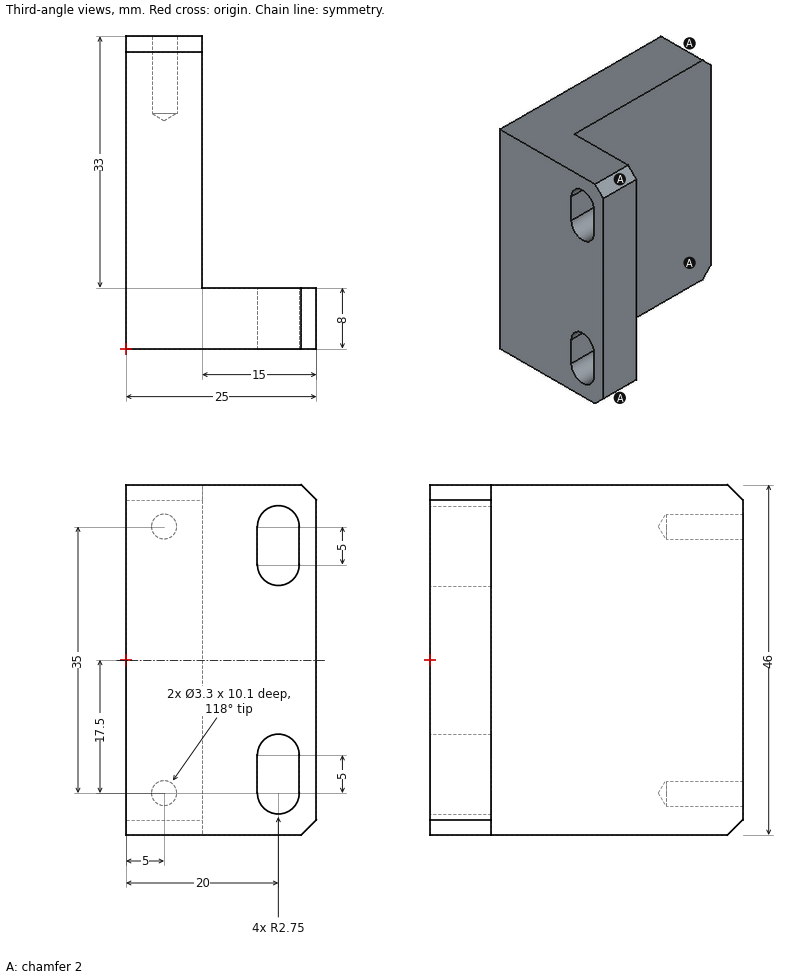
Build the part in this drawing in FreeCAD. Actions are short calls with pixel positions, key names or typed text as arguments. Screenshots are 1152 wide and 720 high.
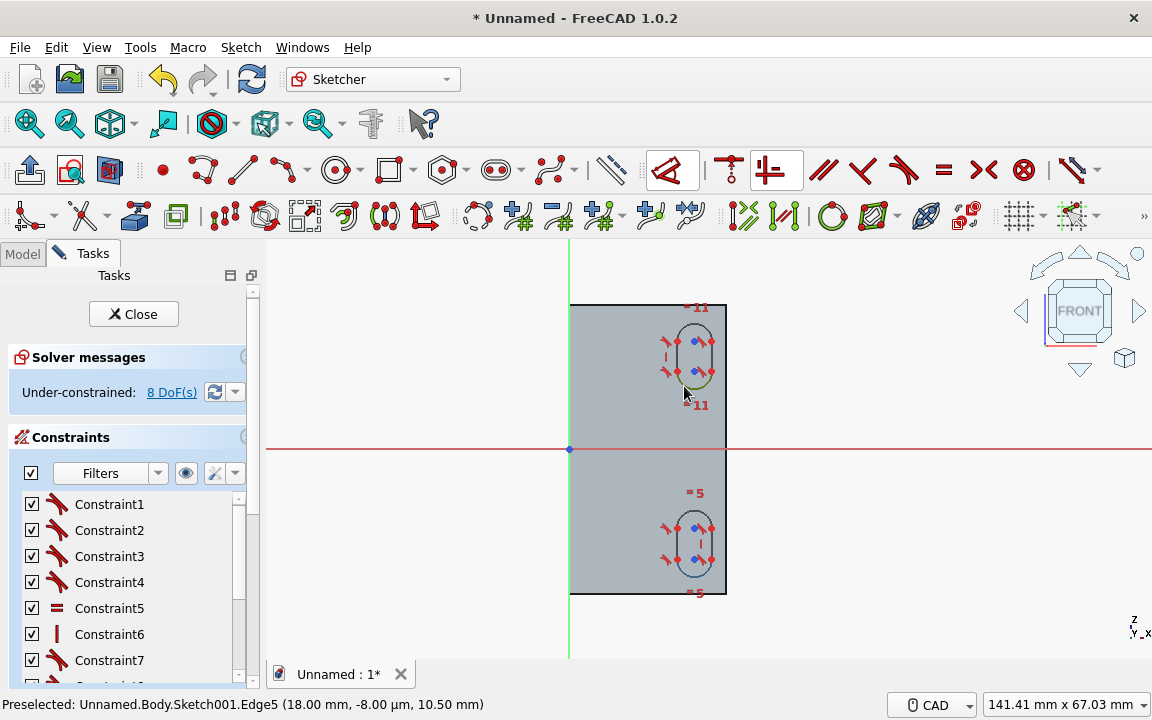
click(944, 170)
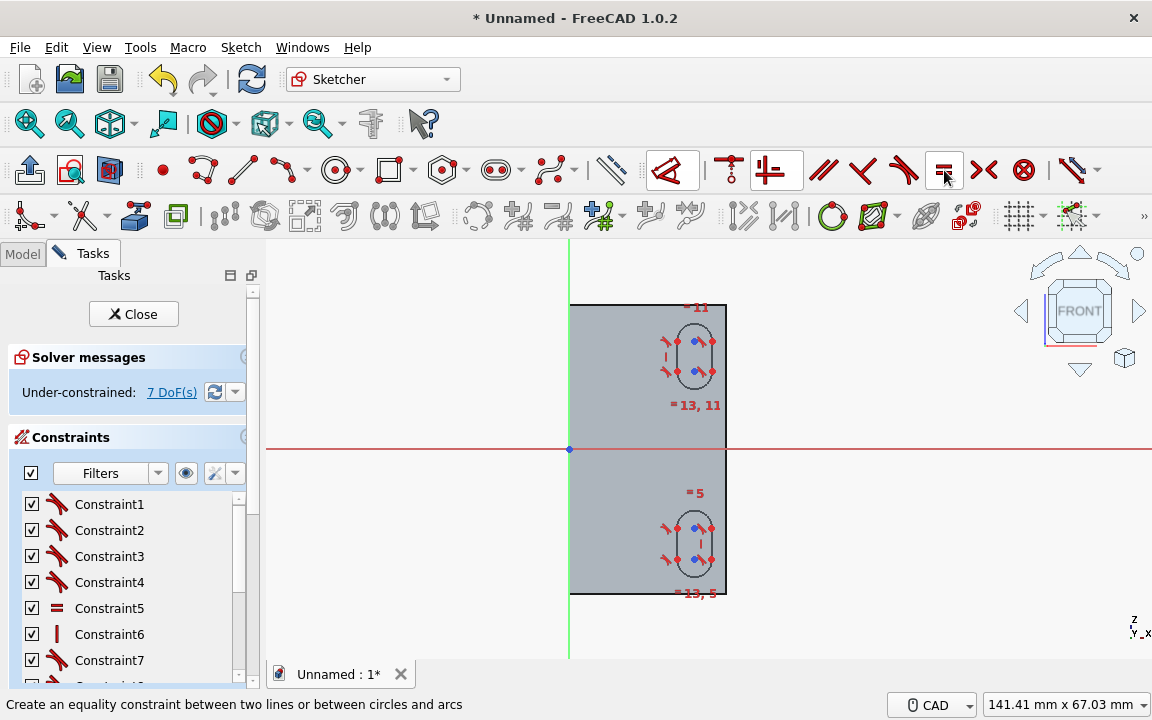
click(695, 528)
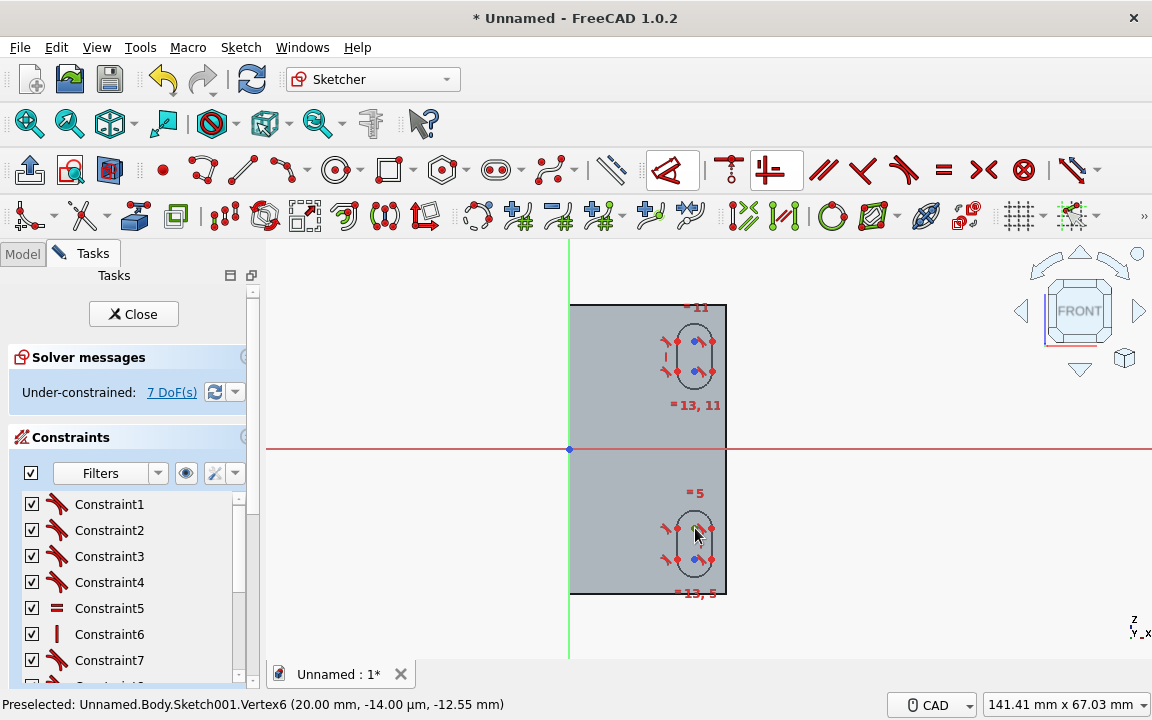
click(695, 372)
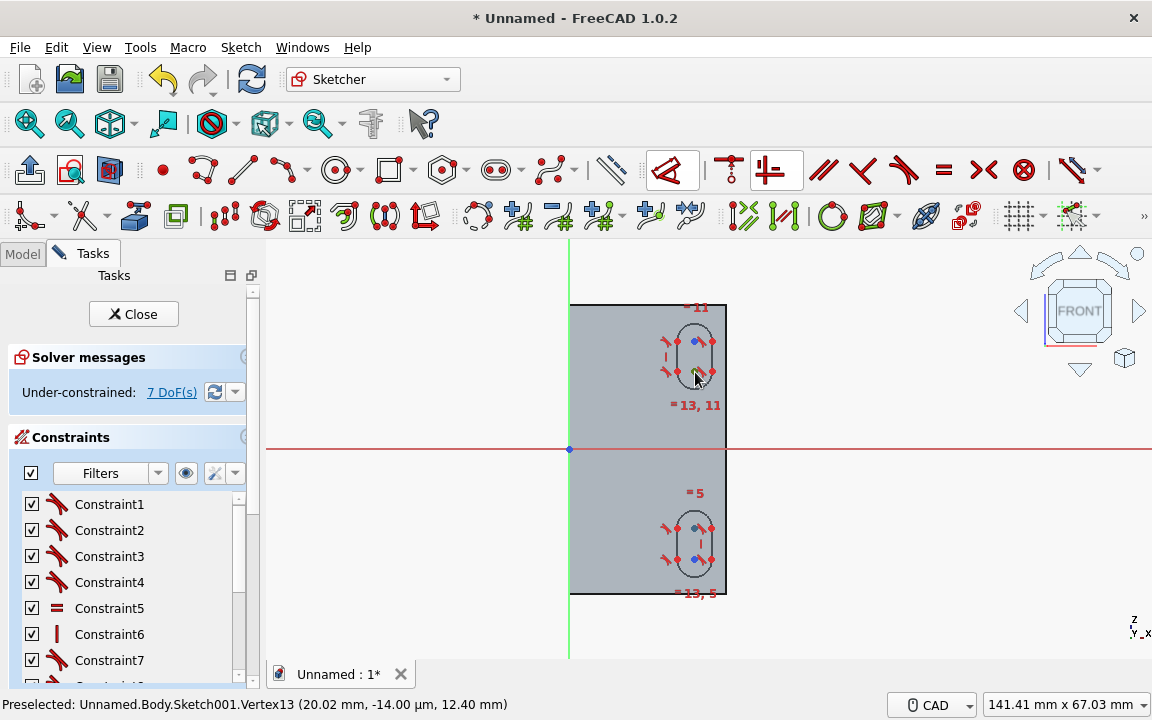
click(344, 449)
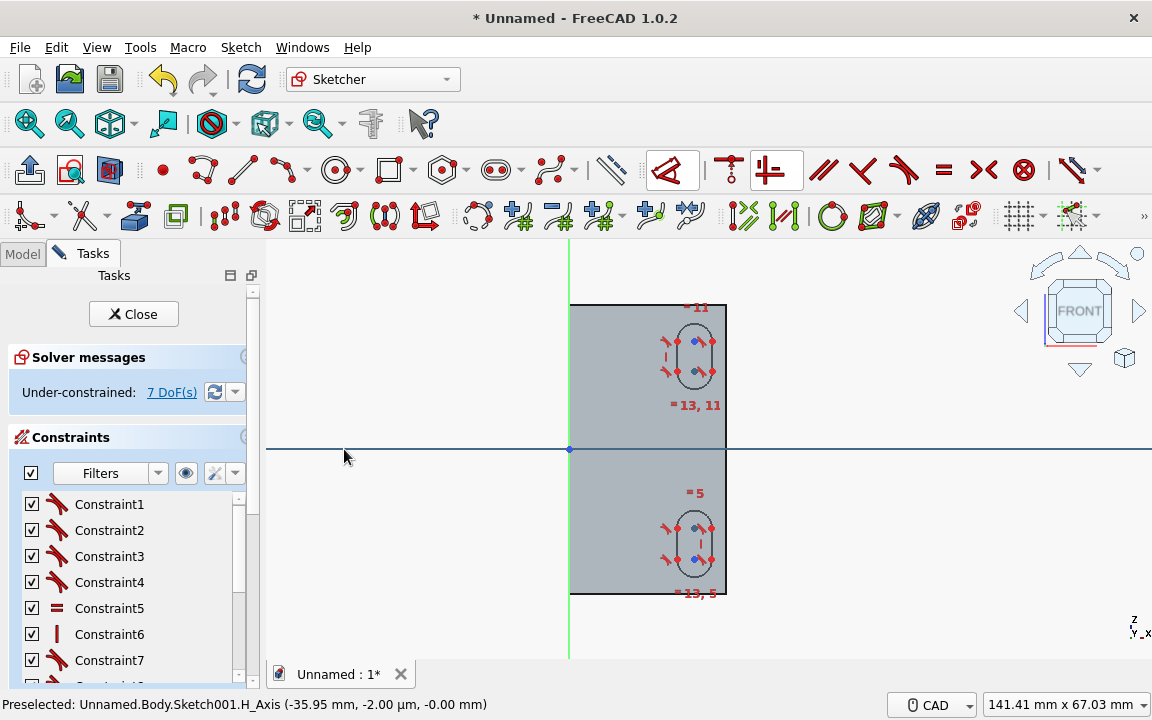
click(984, 170)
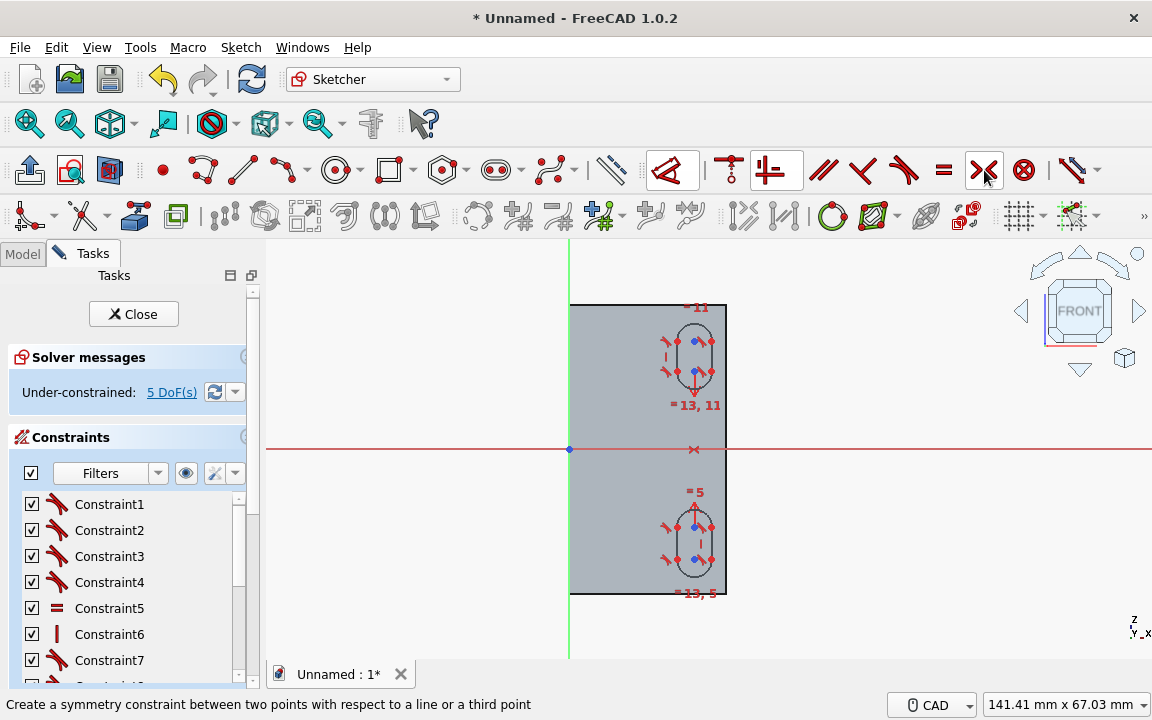
scroll(684, 574, up, 5)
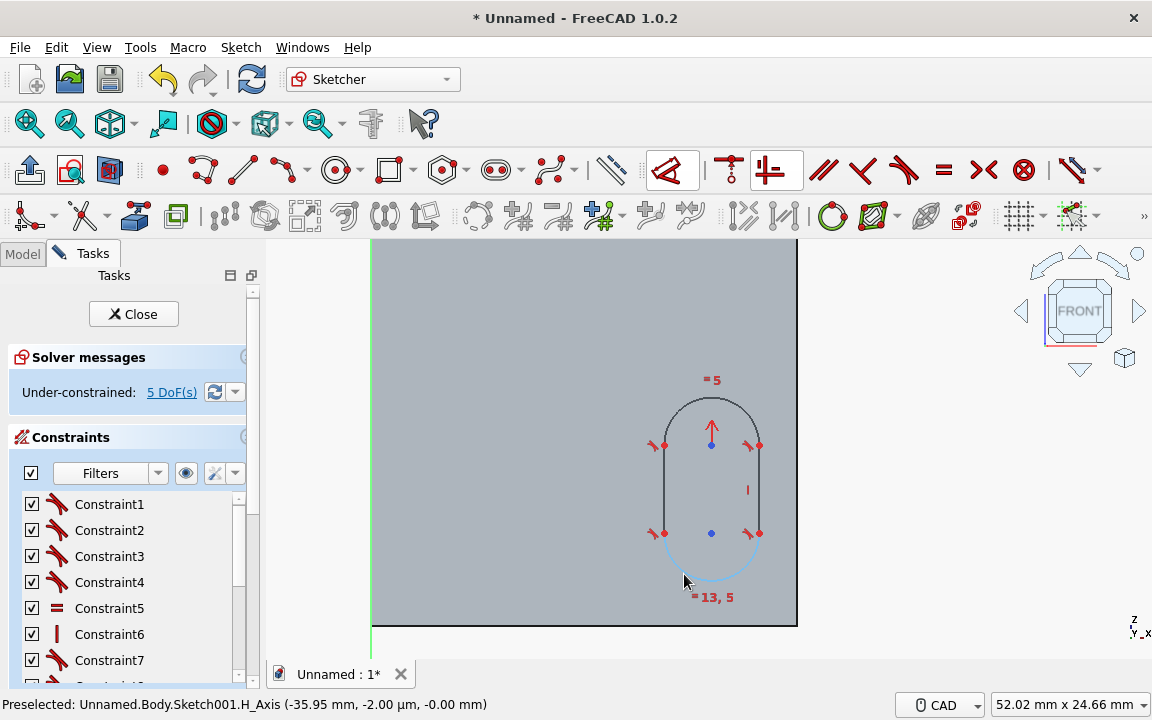
click(684, 572)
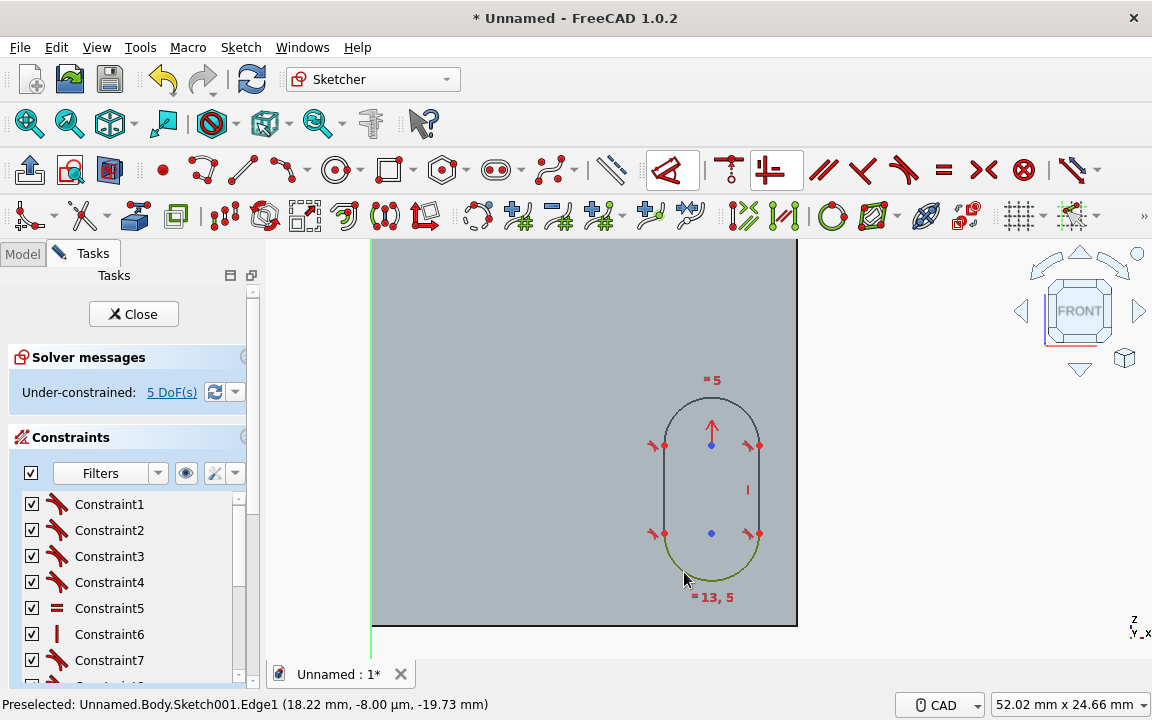
key(k)
key(r)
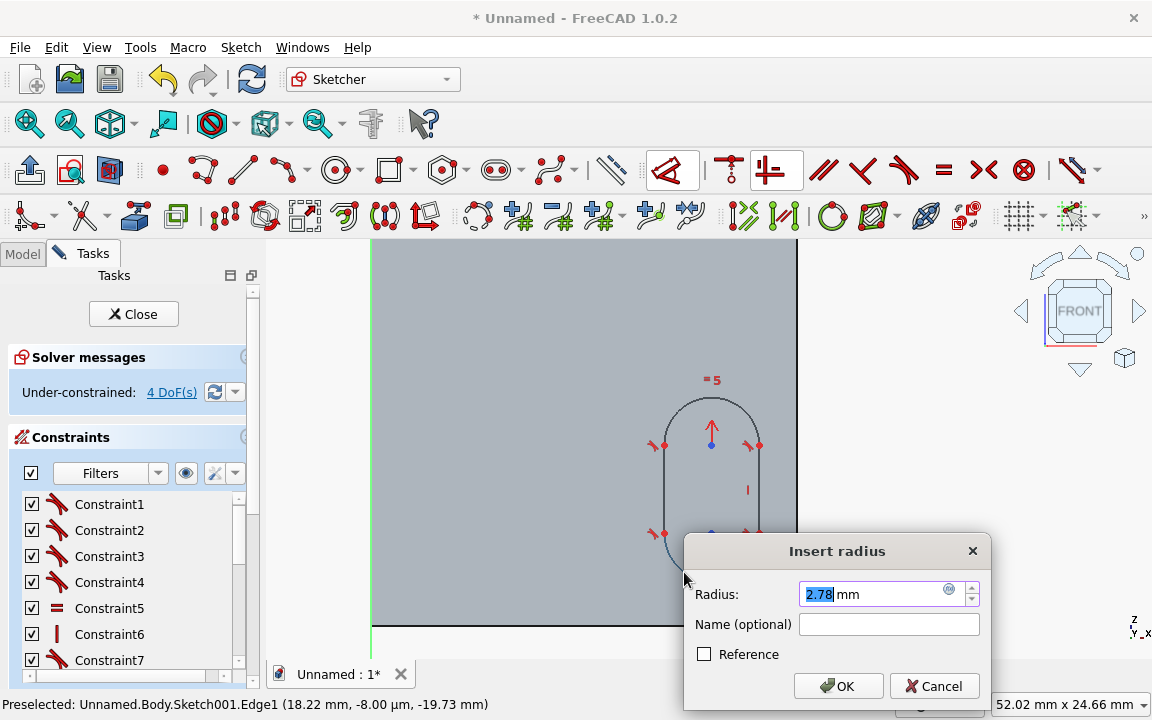
text(2.75)
key(Return)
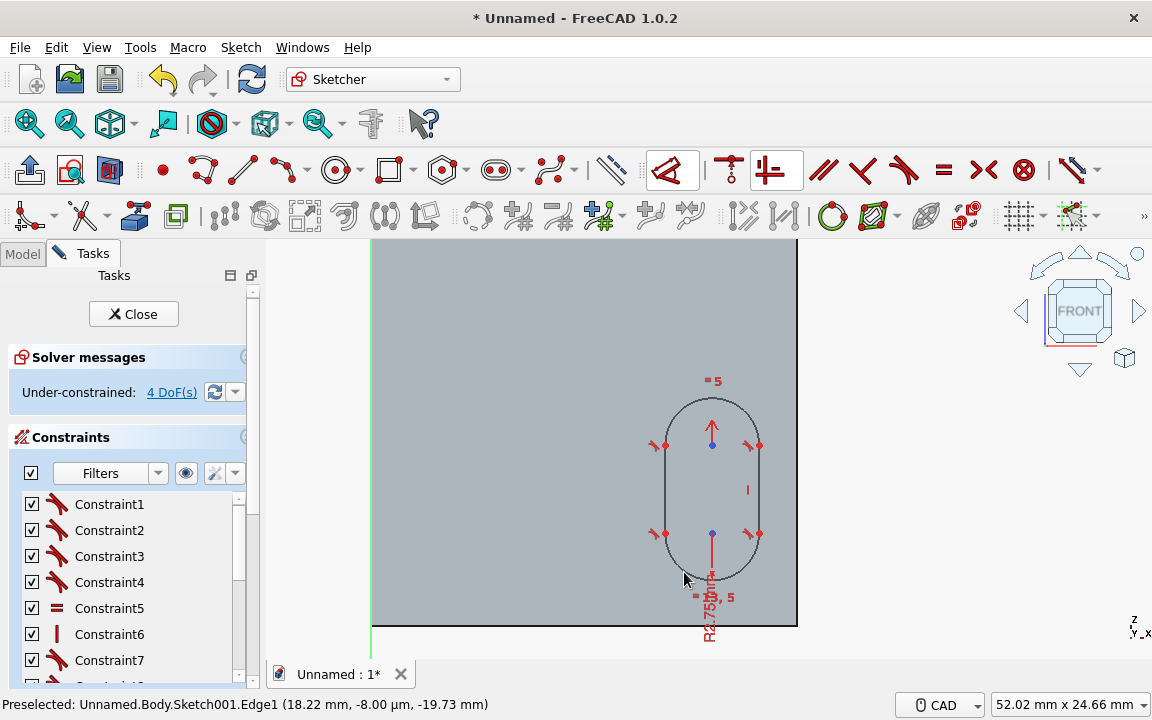
click(665, 507)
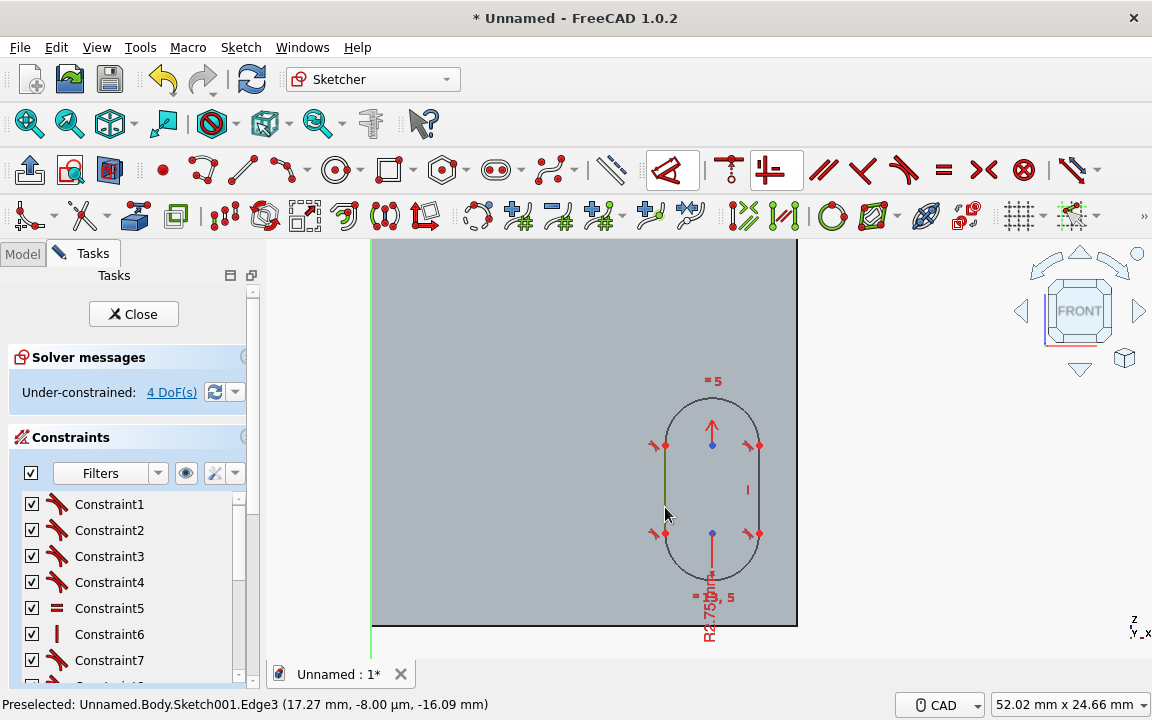
click(694, 170)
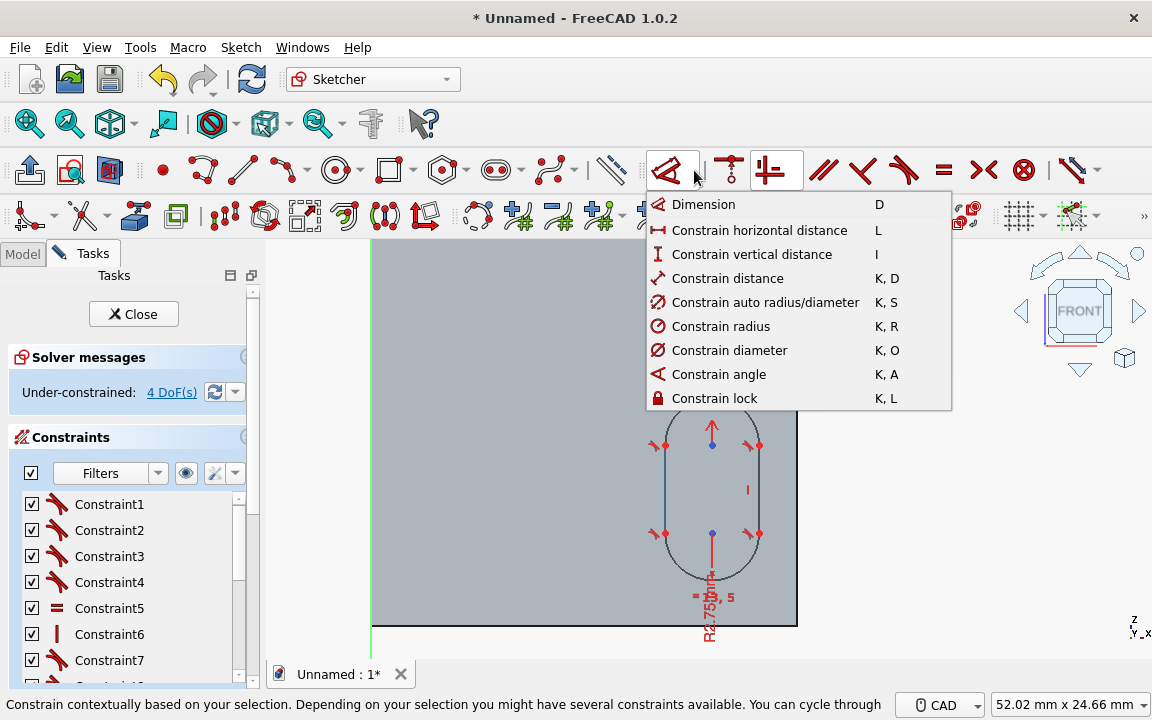
click(799, 254)